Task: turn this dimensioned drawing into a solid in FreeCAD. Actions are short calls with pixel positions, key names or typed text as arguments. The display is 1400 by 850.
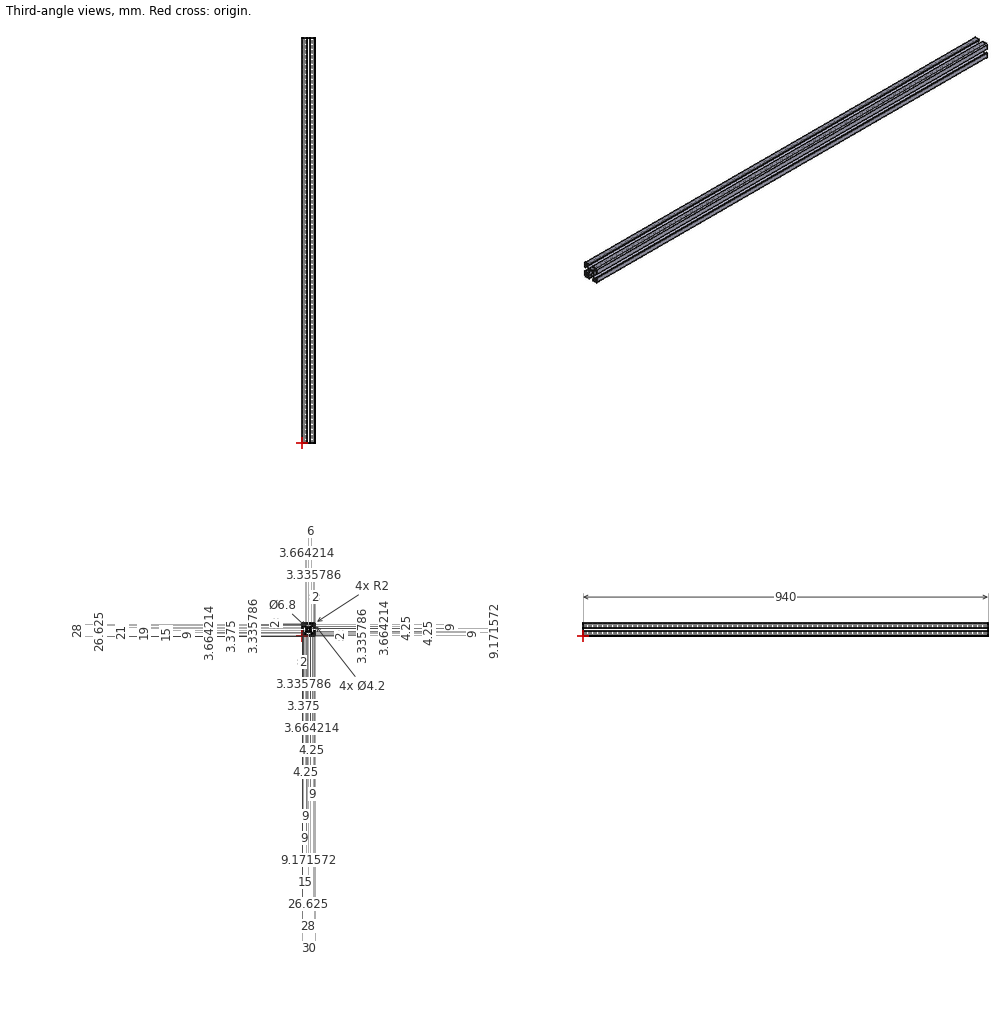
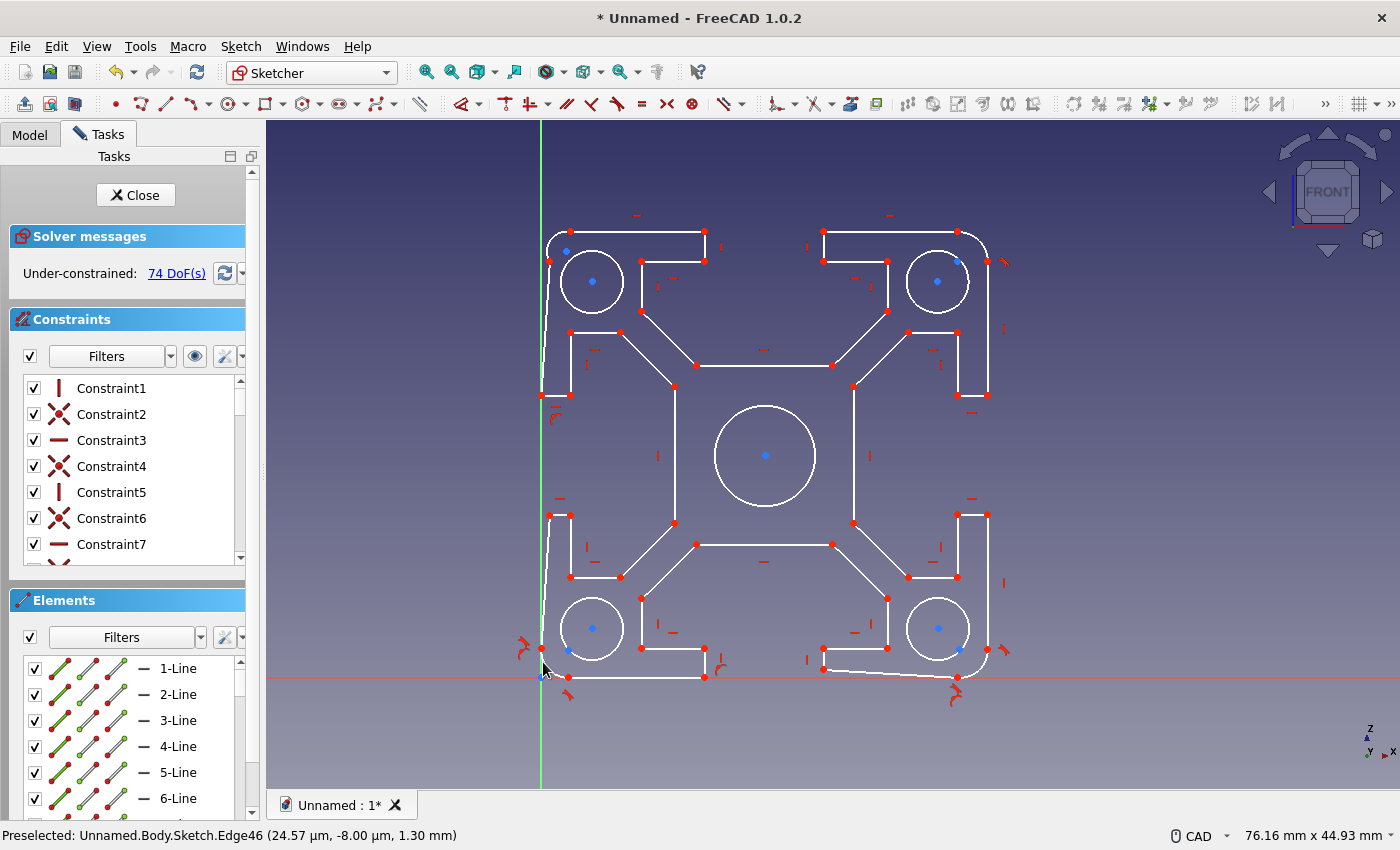
click(544, 356)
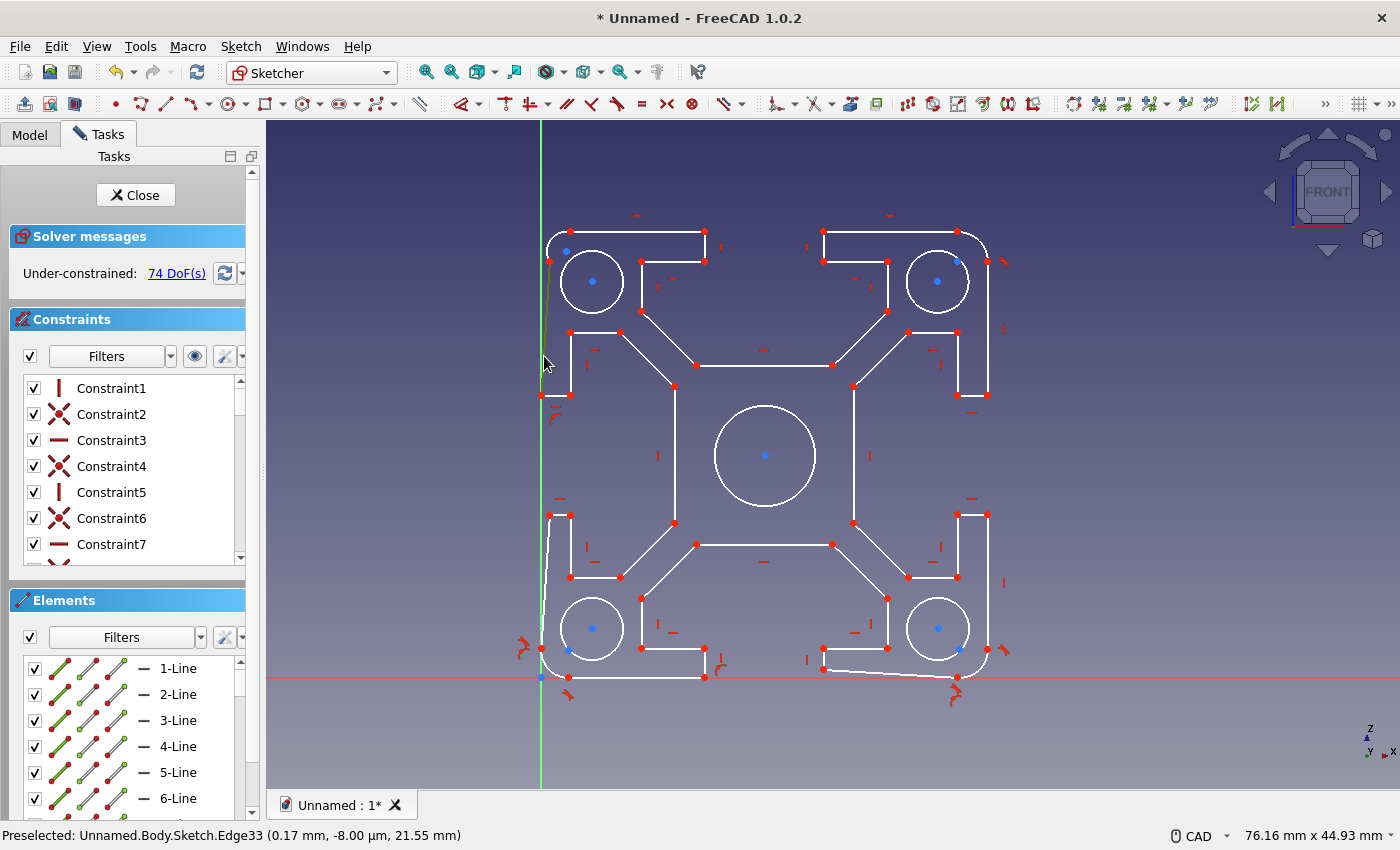
click(557, 234)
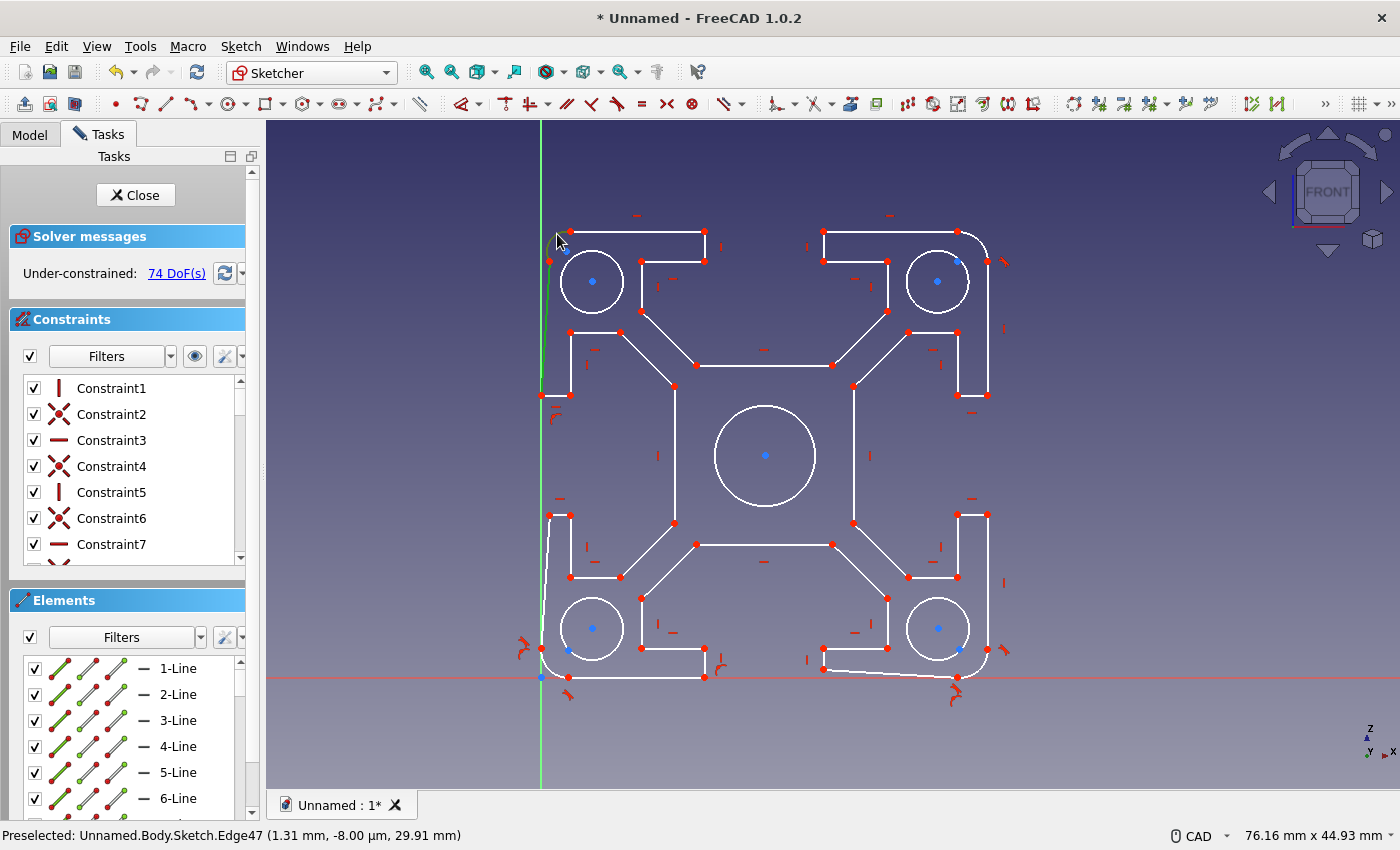
key(t)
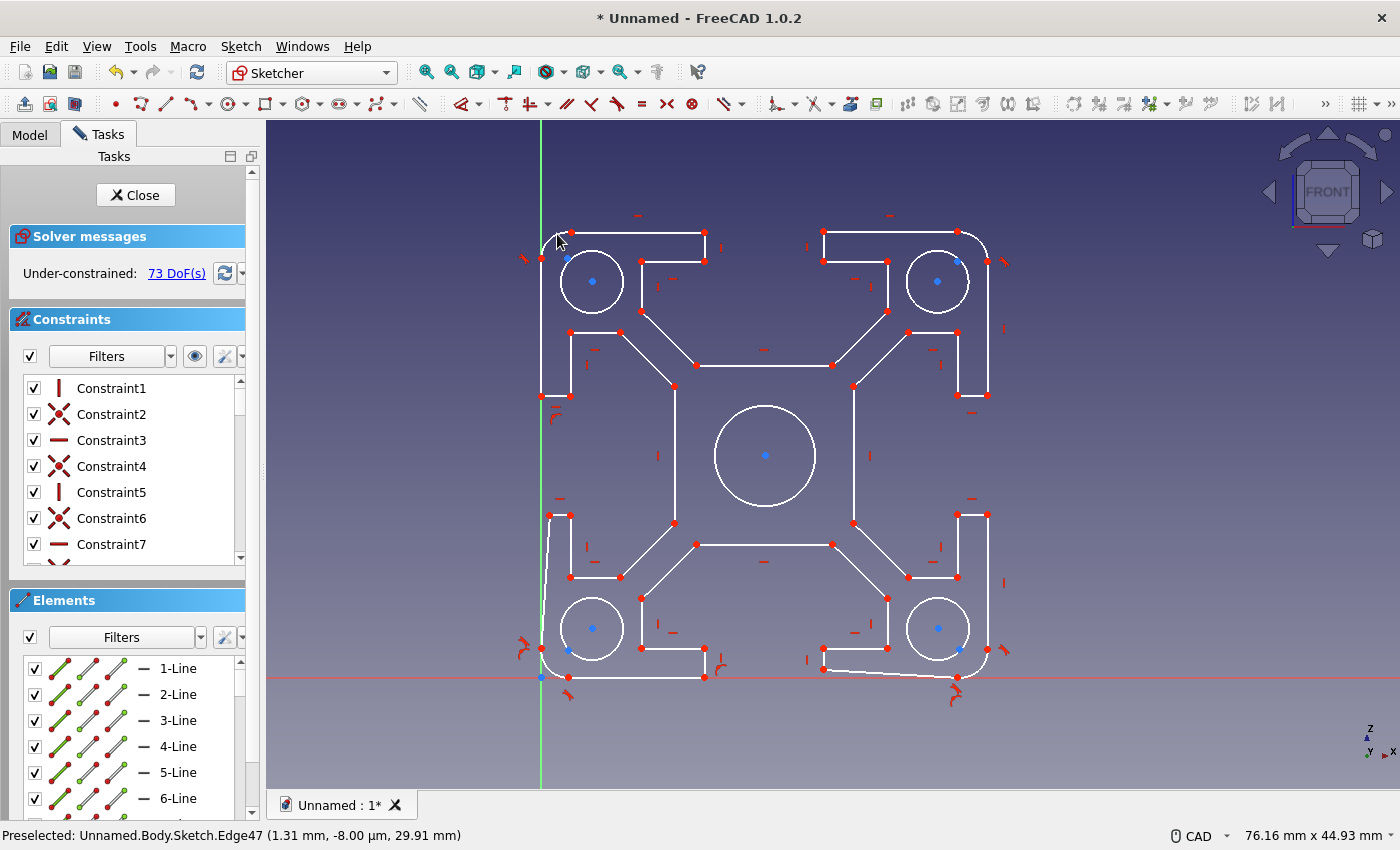
click(611, 233)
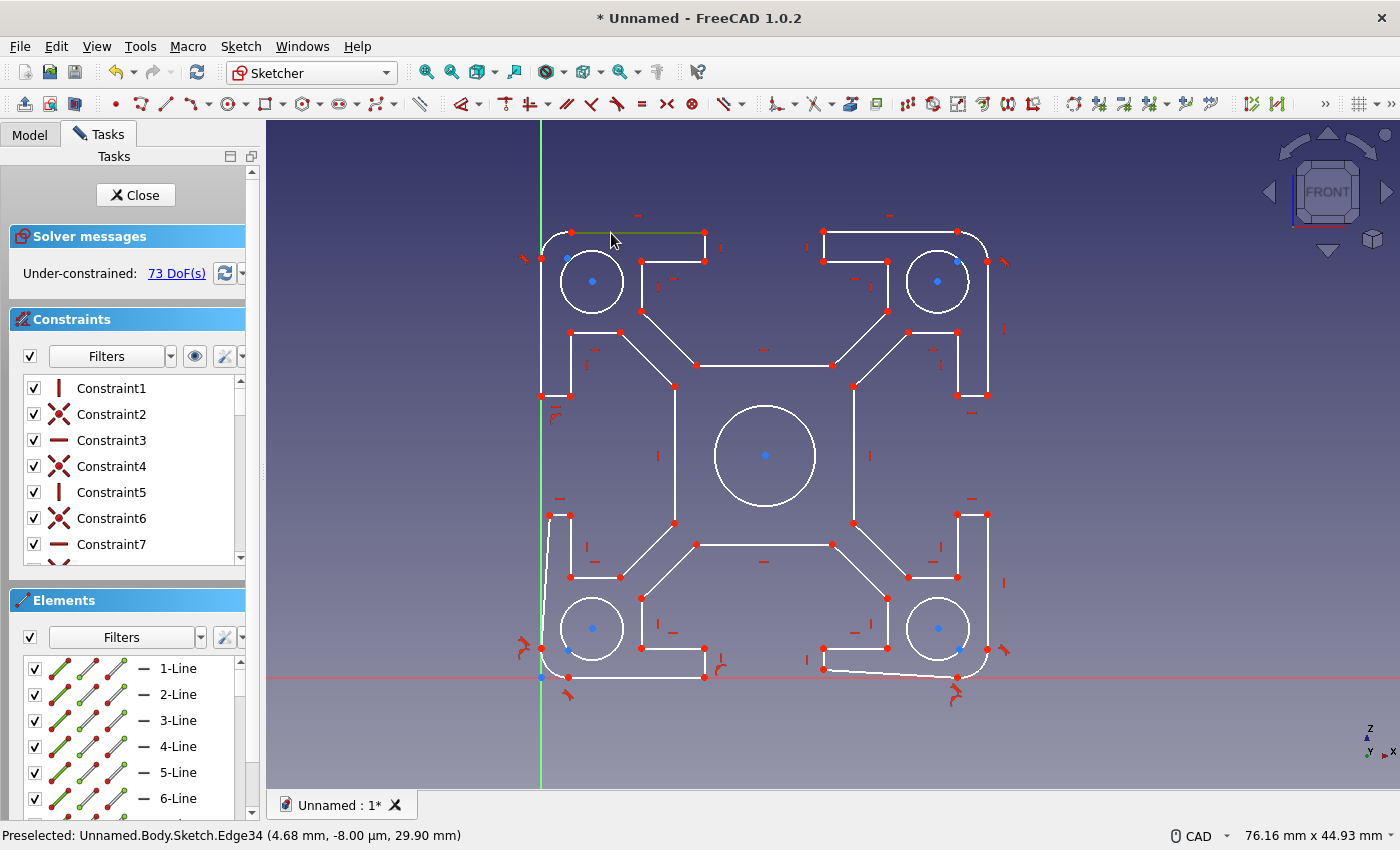
click(558, 234)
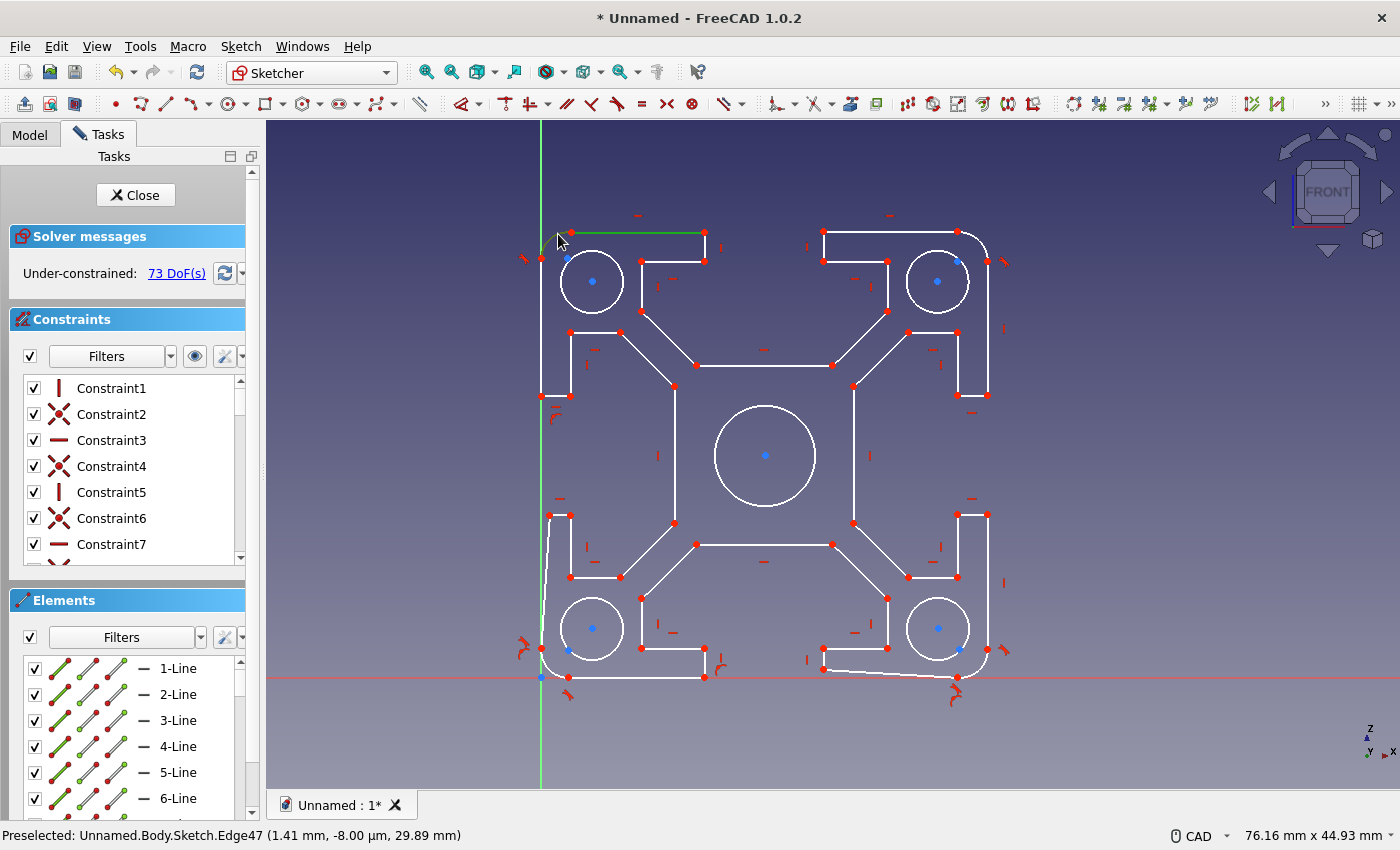
key(t)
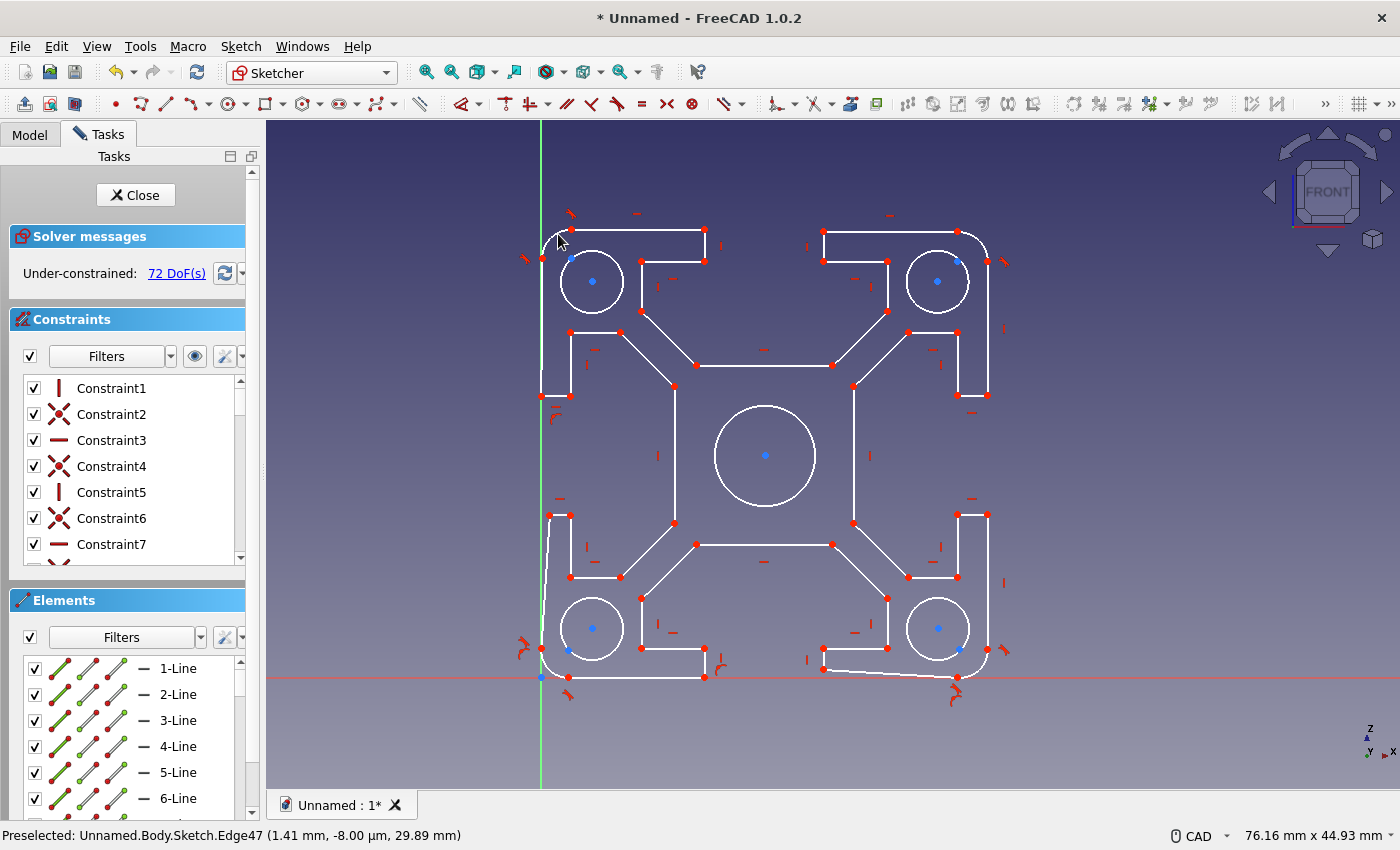
click(864, 232)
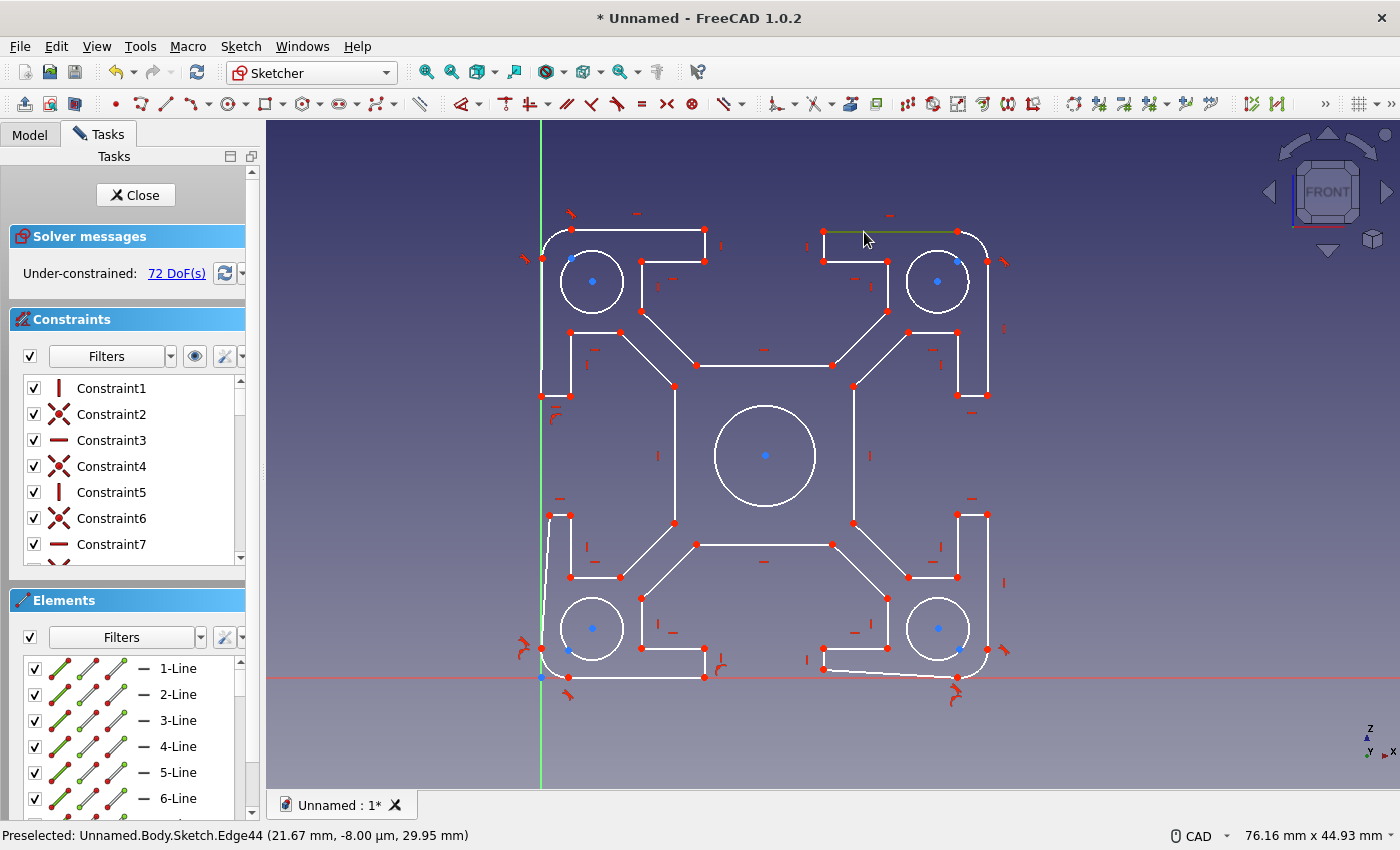
click(985, 248)